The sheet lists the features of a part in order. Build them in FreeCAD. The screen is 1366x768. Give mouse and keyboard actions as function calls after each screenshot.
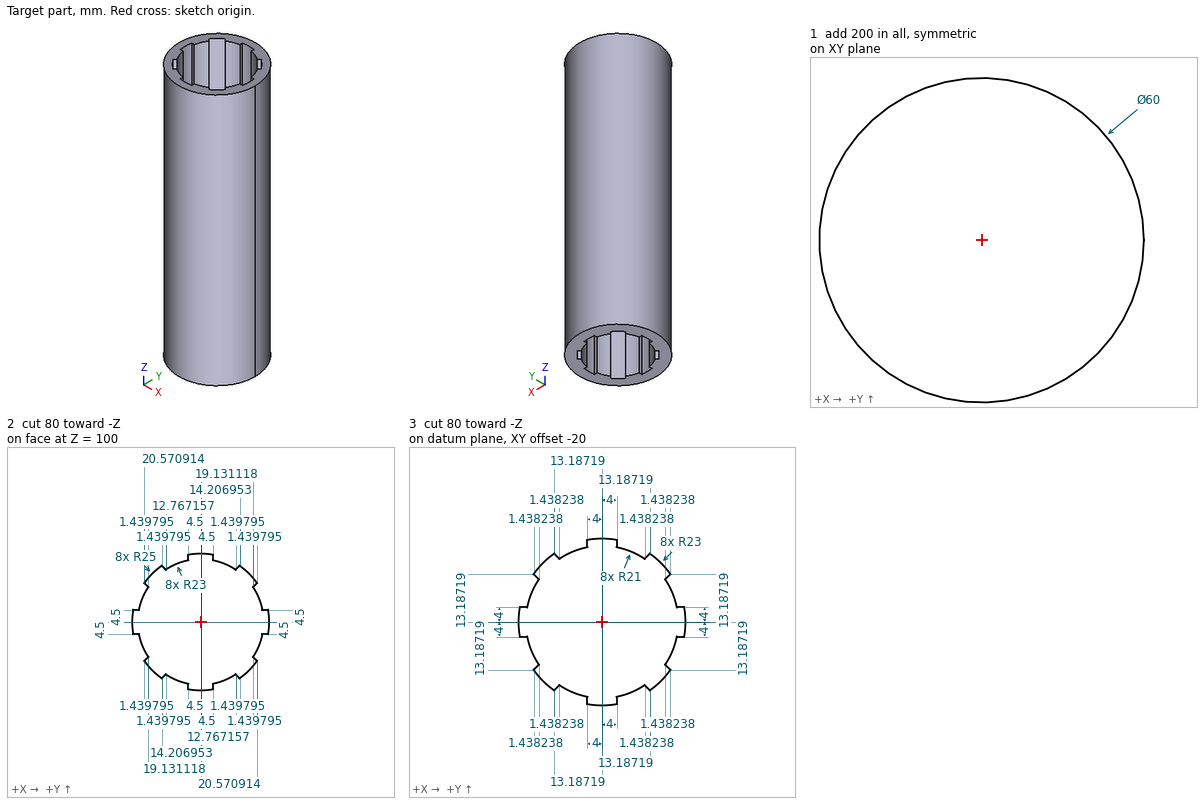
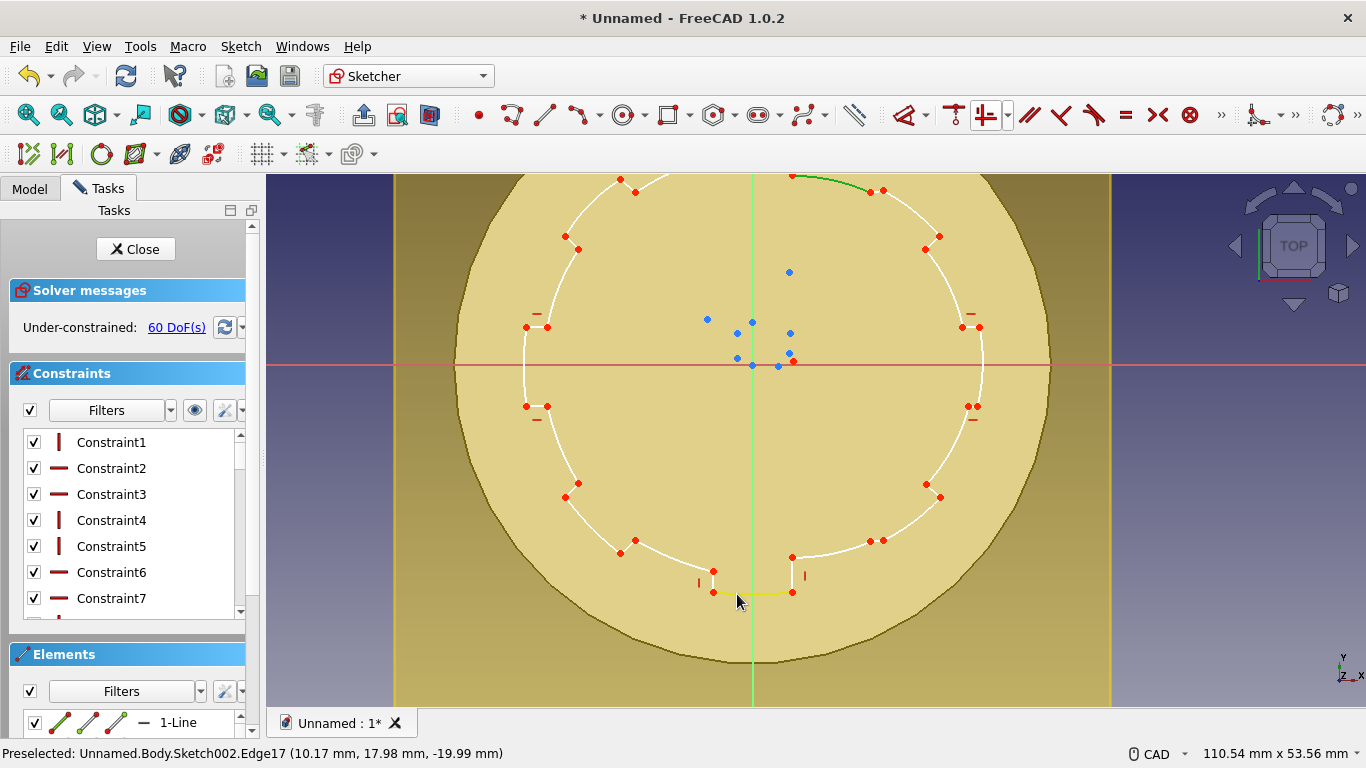
click(737, 594)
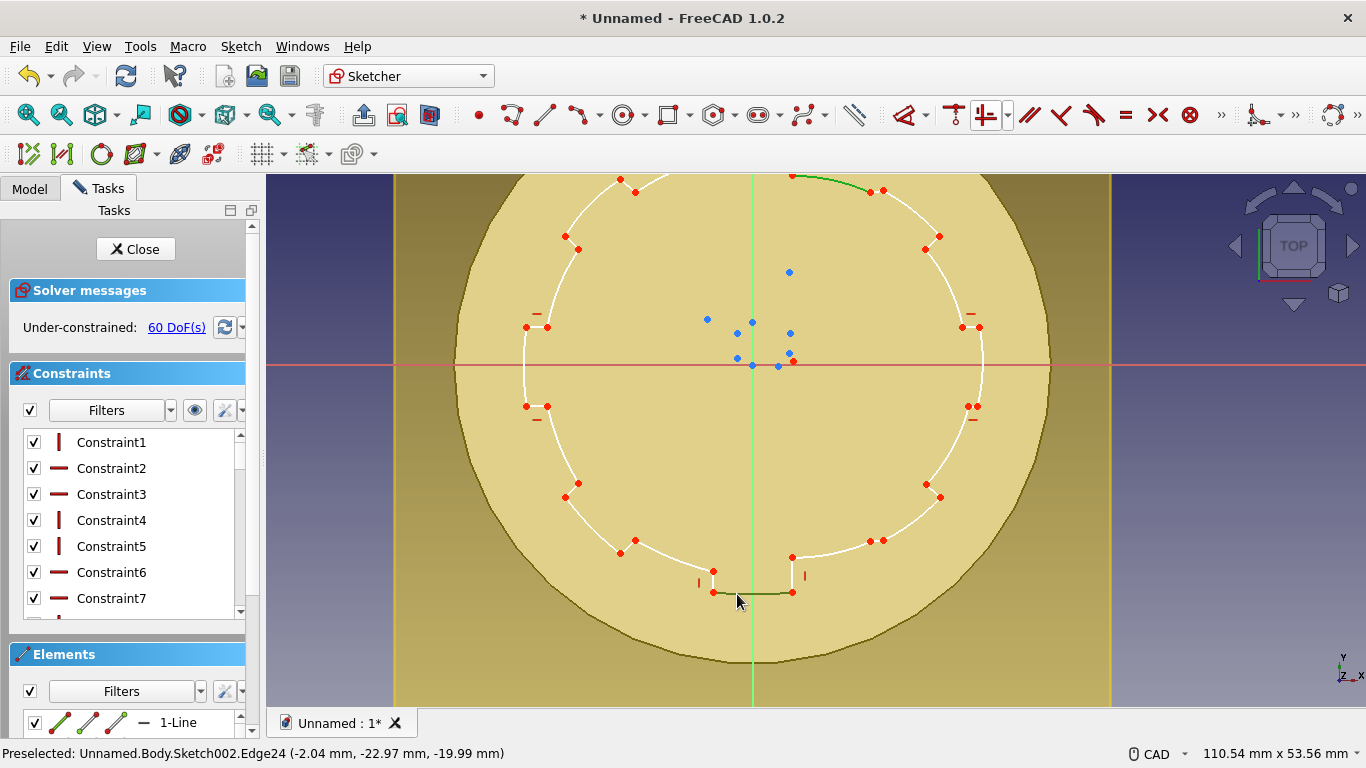
click(954, 116)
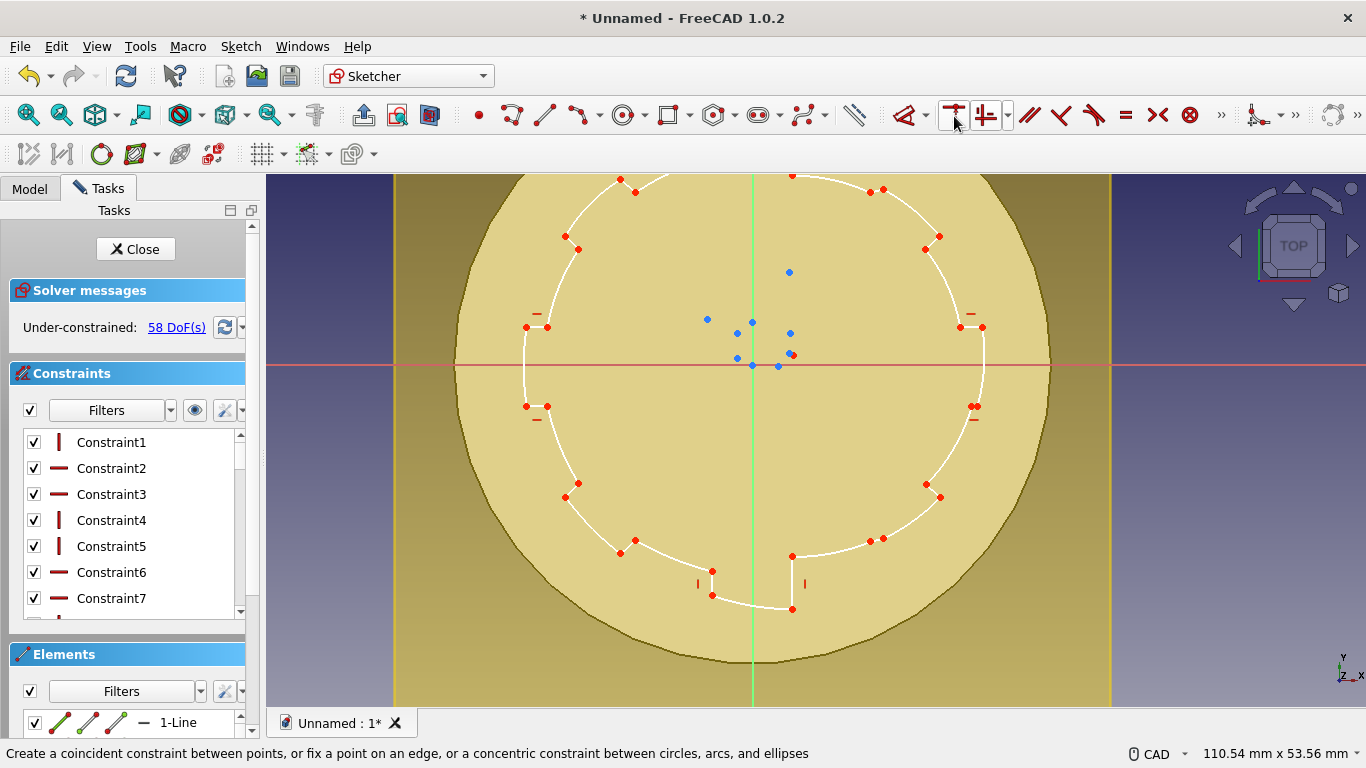
scroll(737, 594, down, 2)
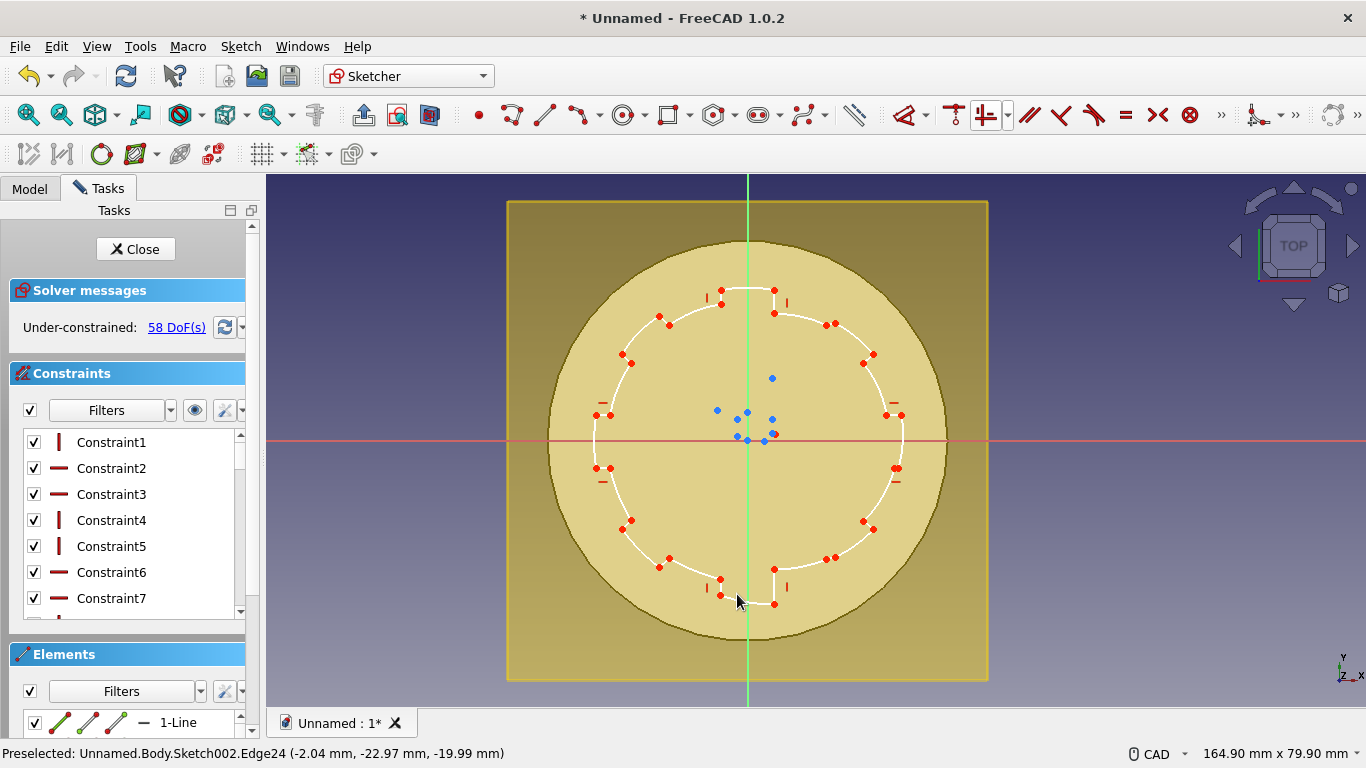
click(811, 319)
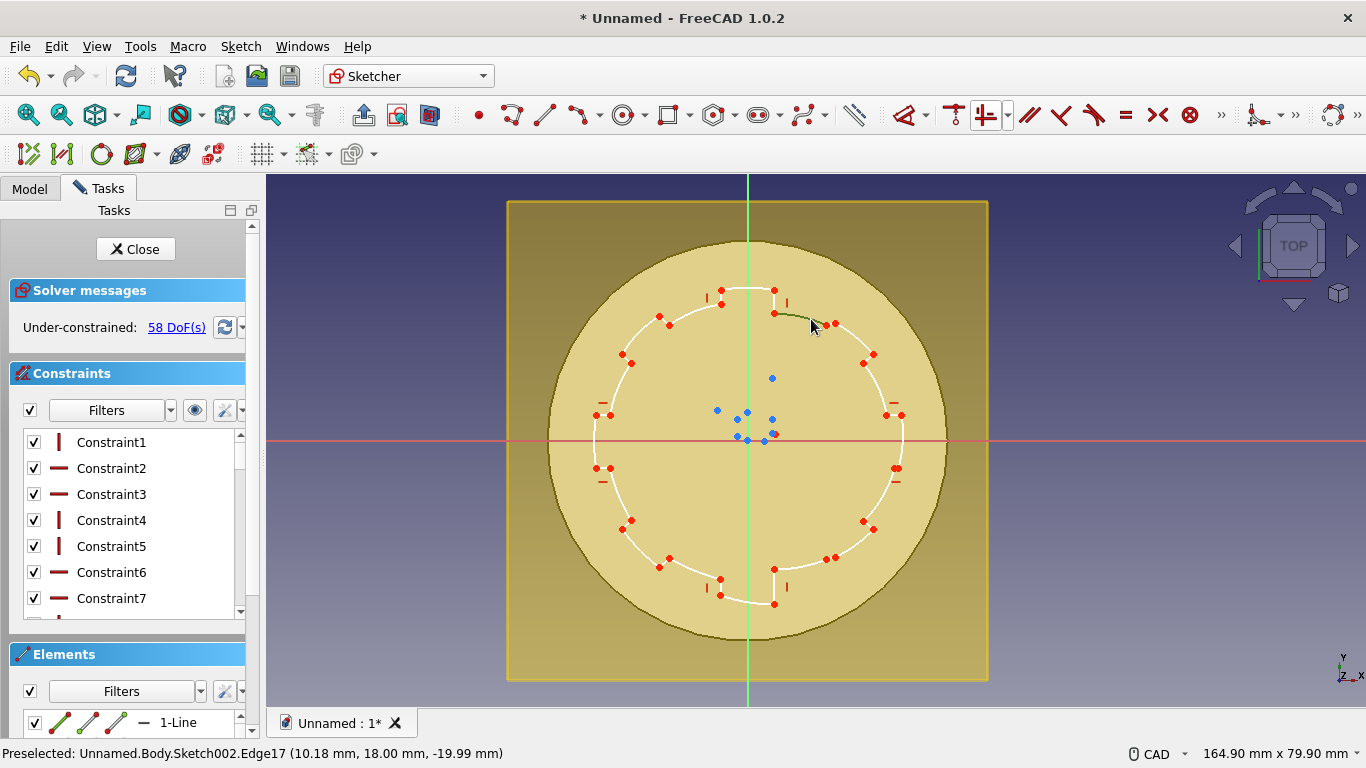
click(684, 566)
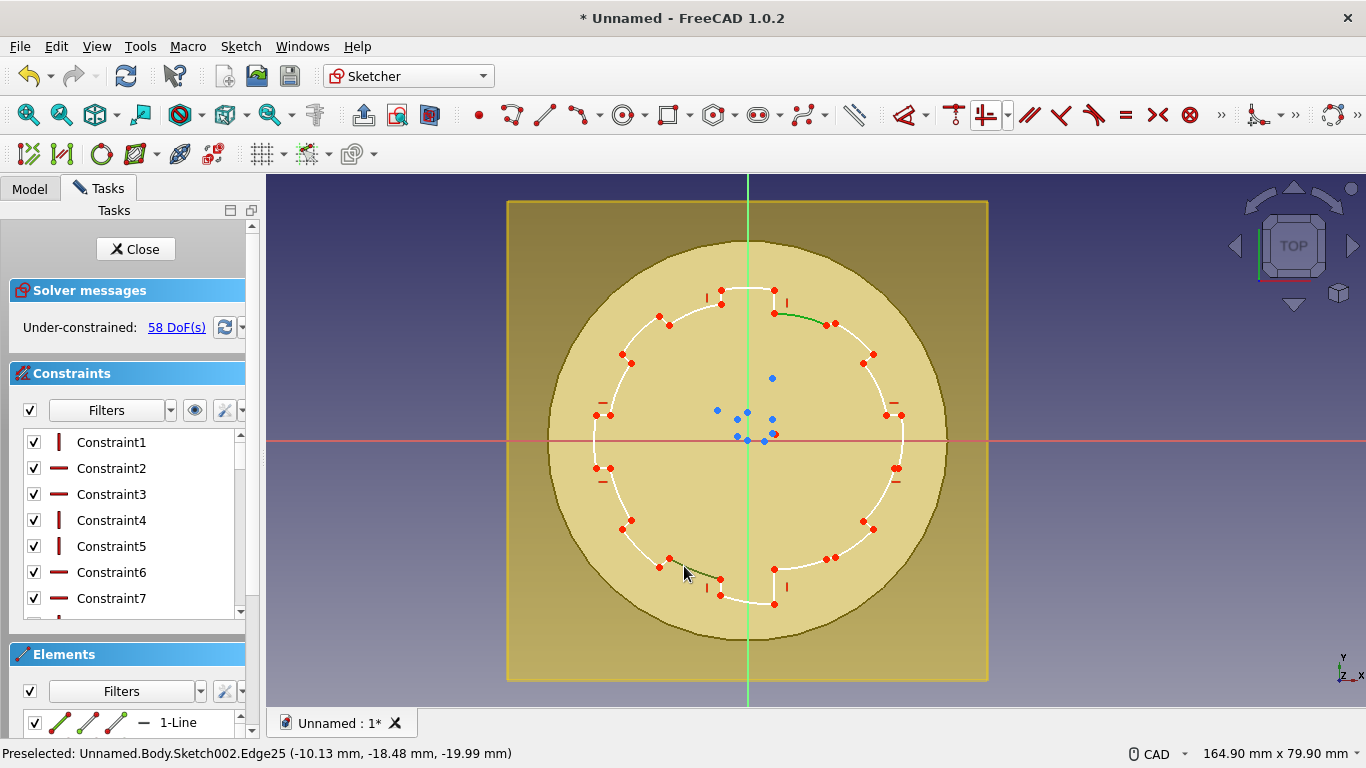
click(954, 116)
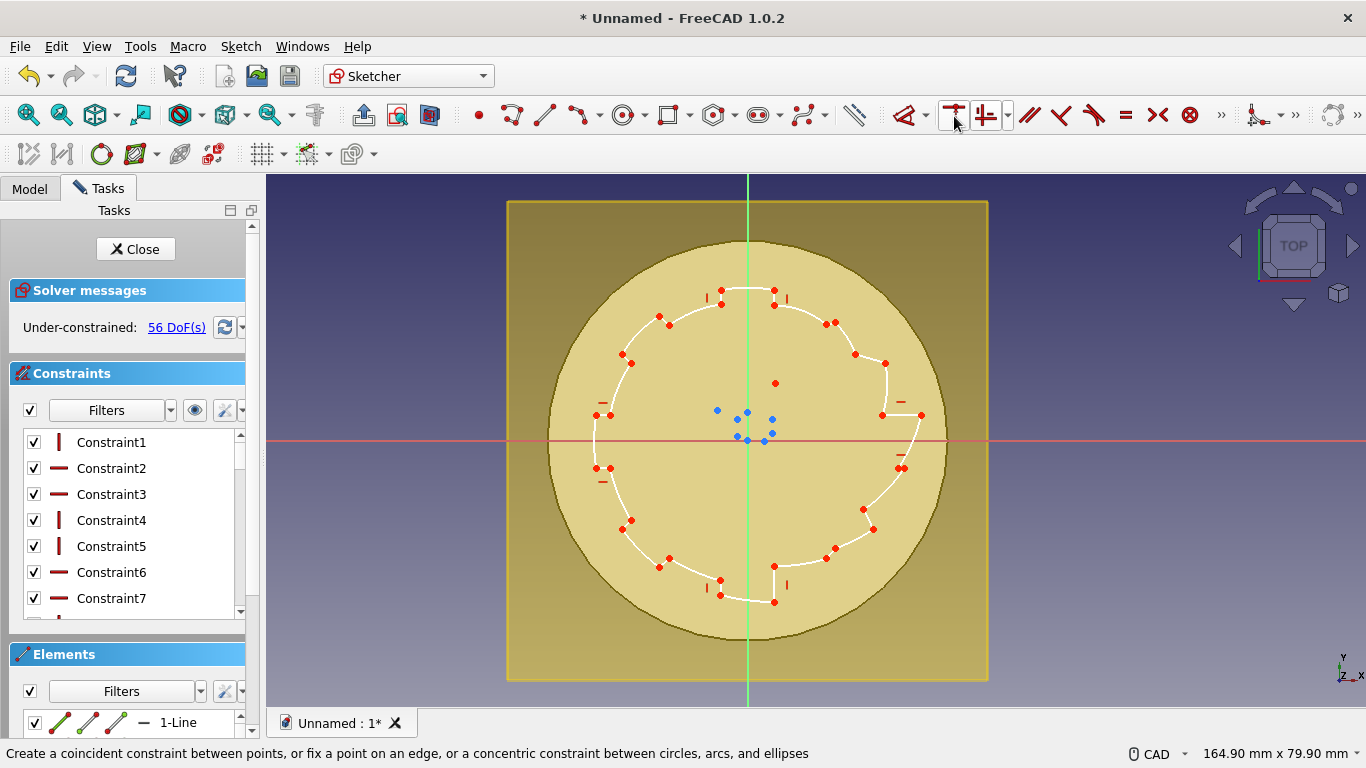
click(813, 315)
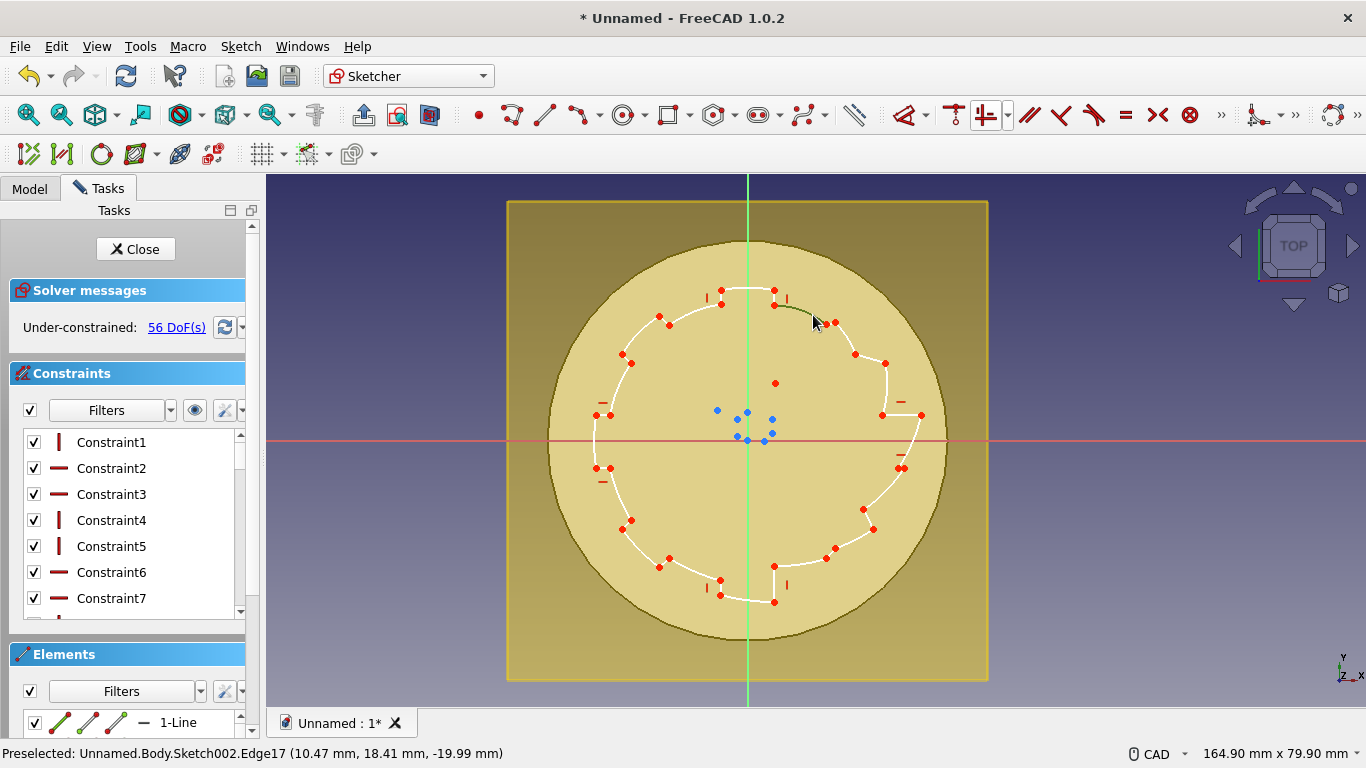
click(632, 542)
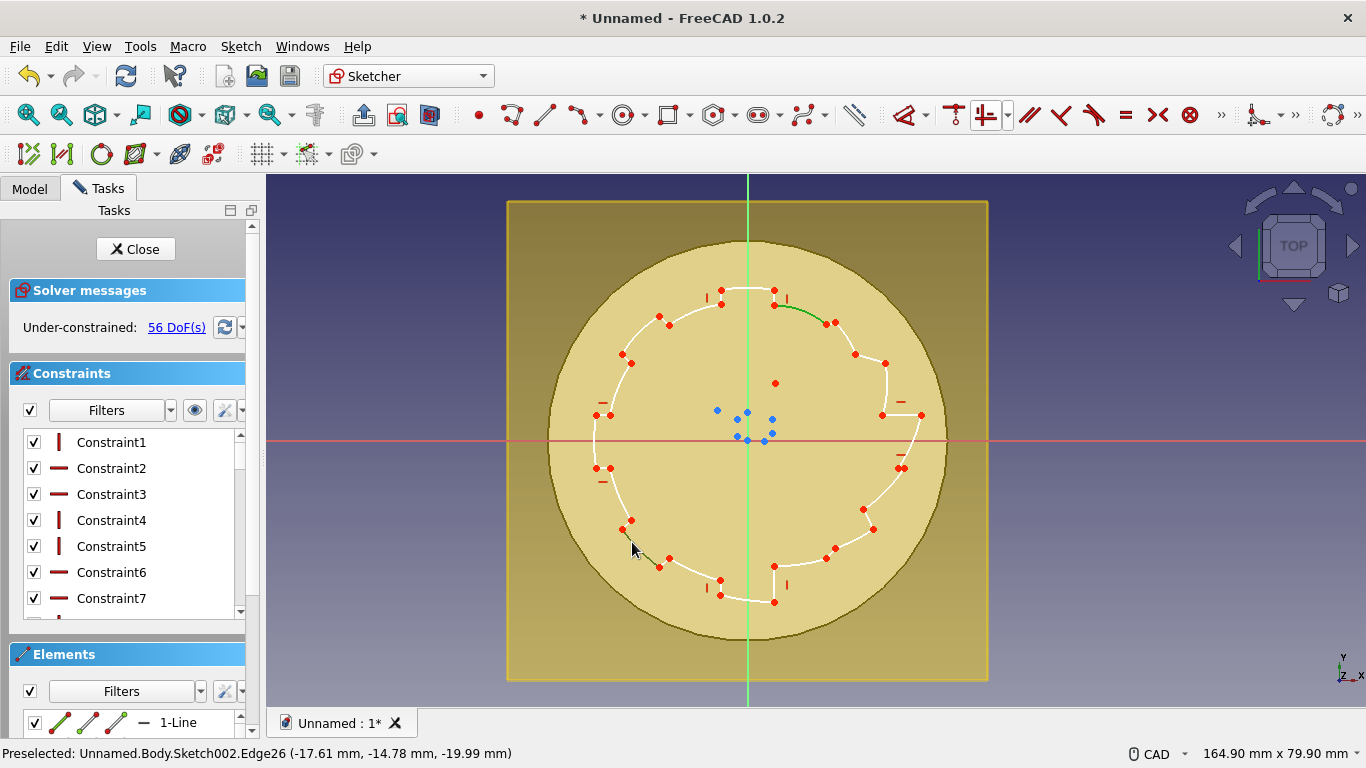
click(954, 116)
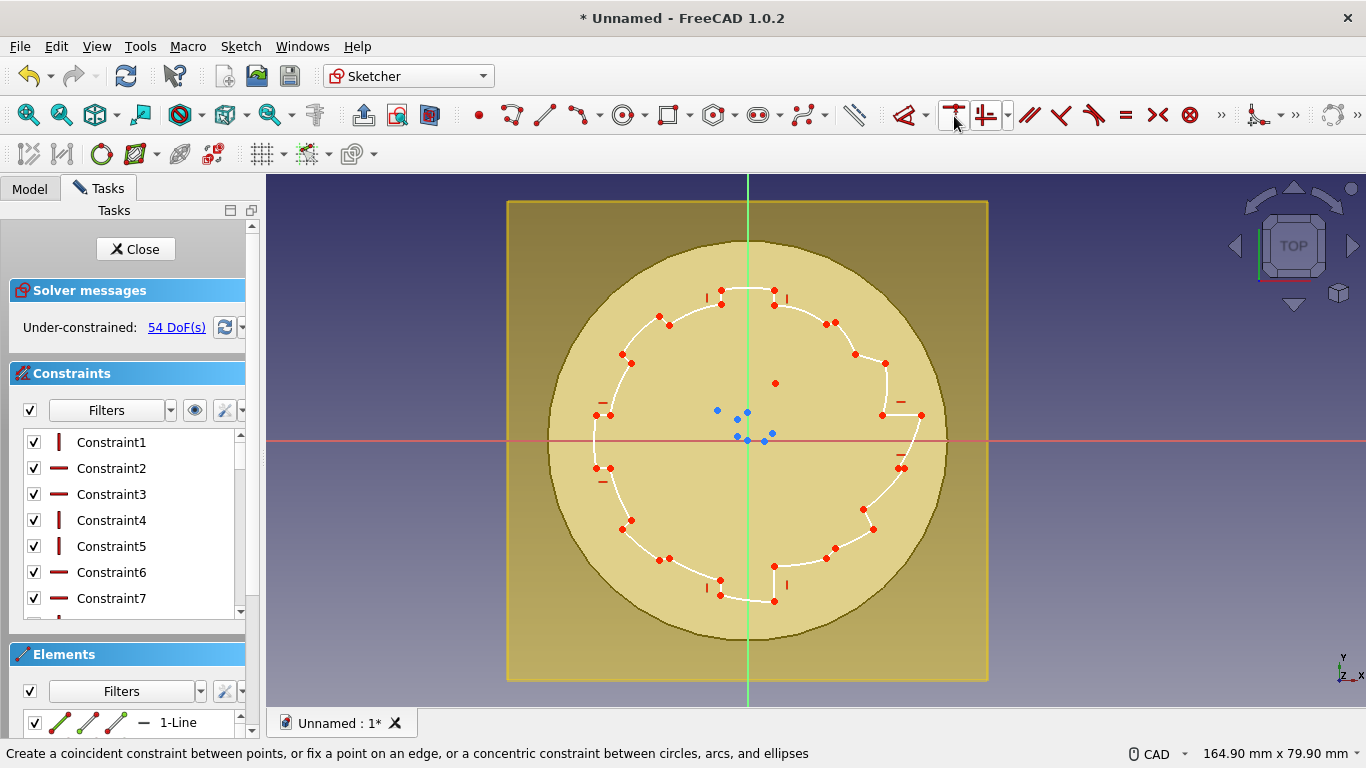
click(813, 315)